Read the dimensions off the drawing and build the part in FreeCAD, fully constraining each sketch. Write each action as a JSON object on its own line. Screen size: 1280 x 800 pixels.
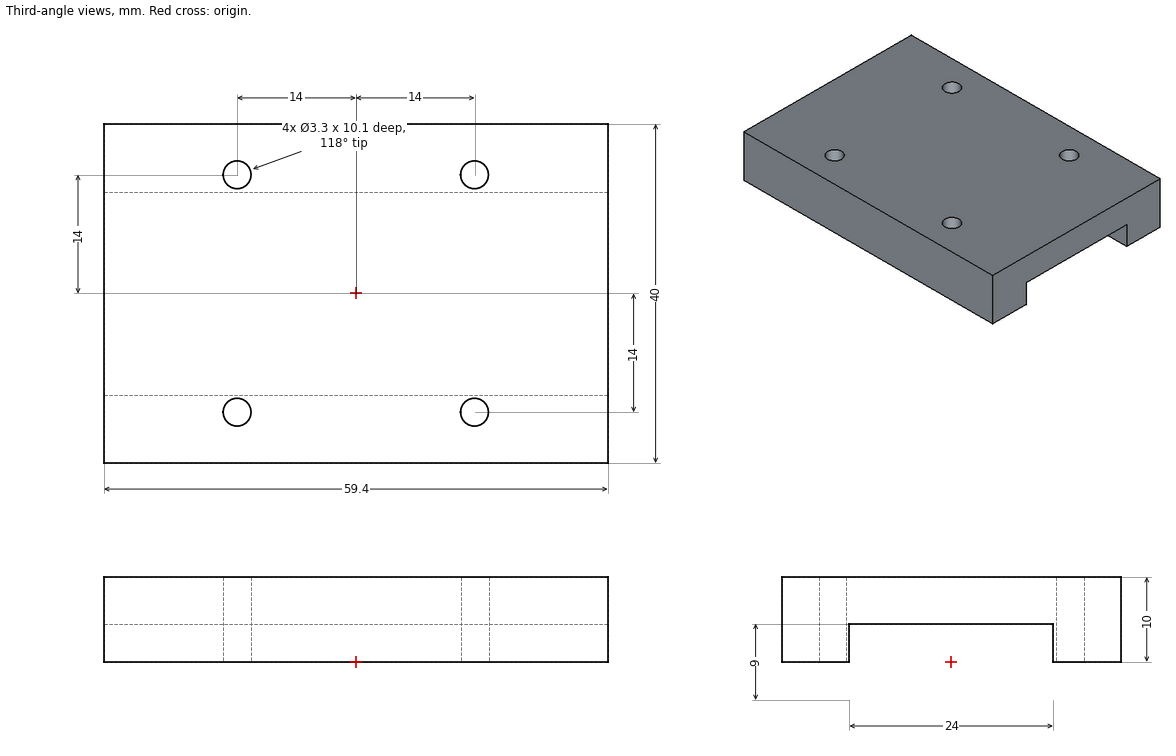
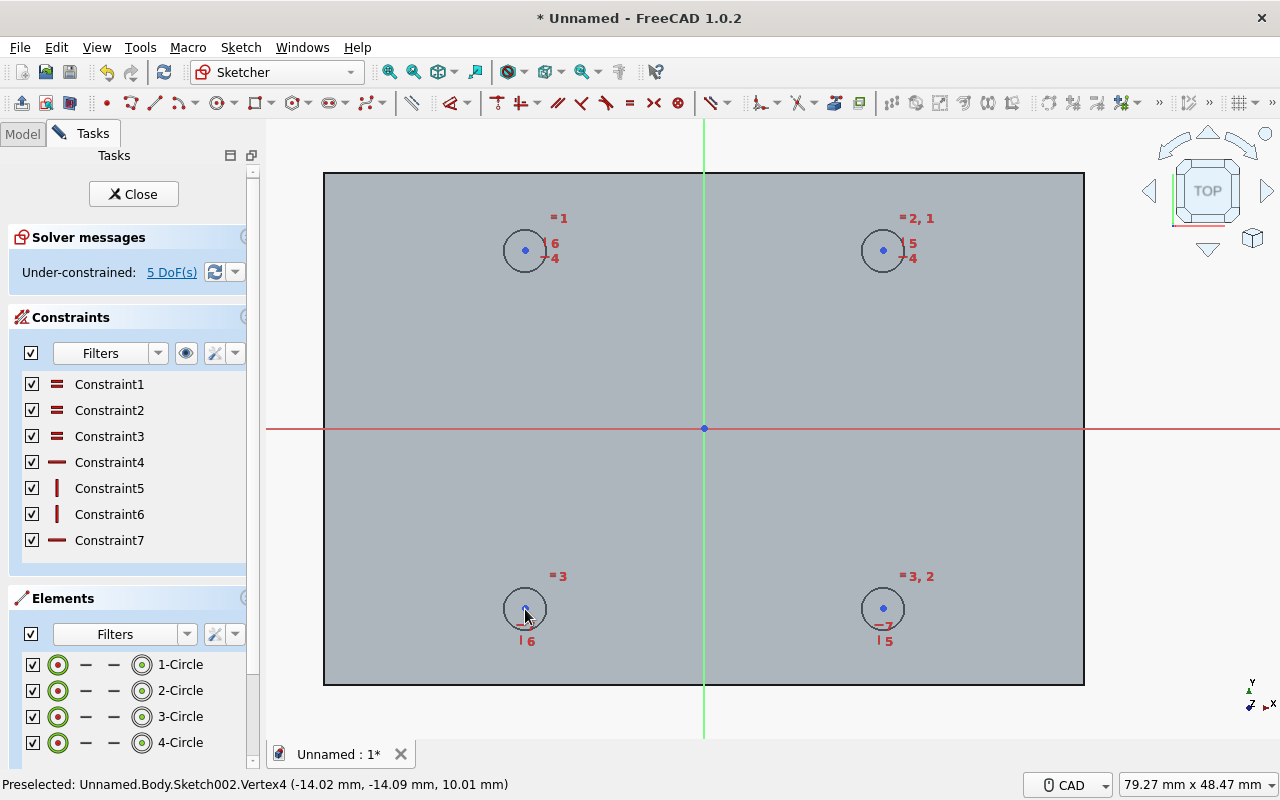
{"action": "key", "text": "d"}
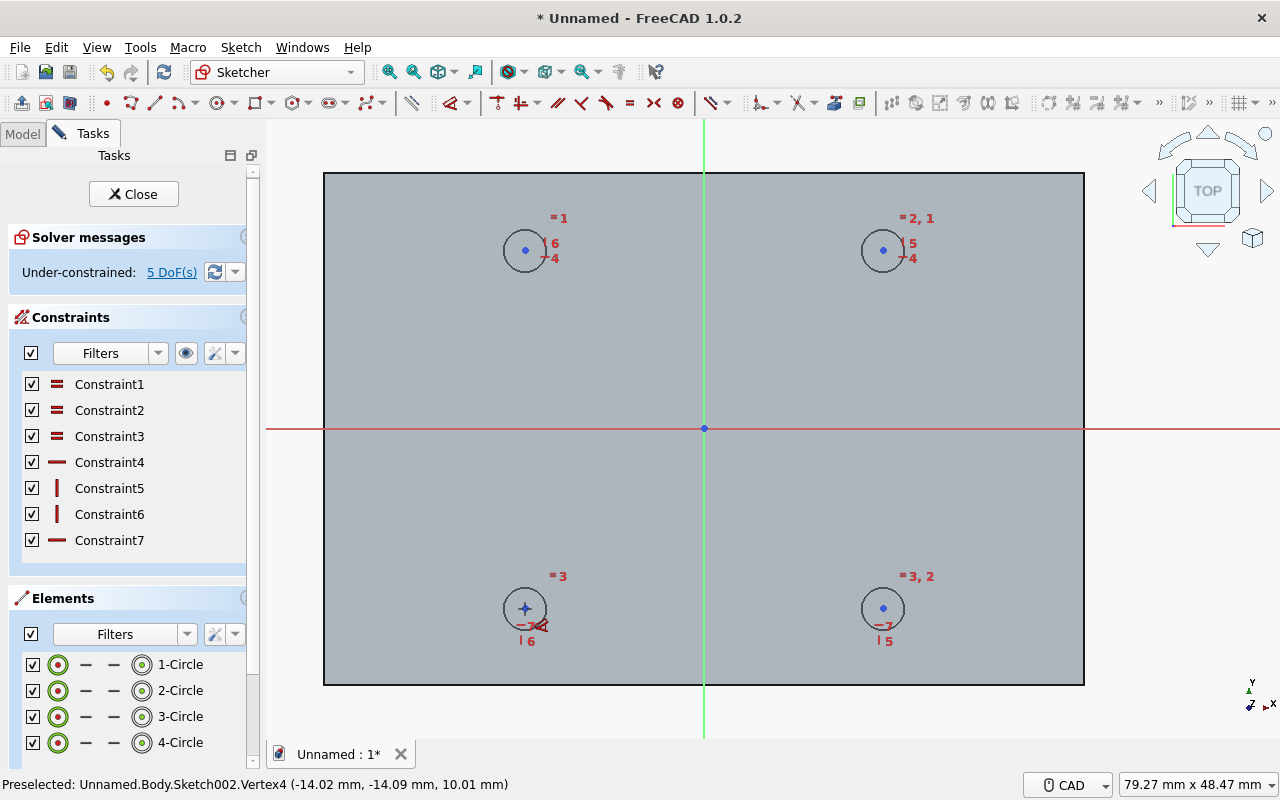
{"action": "left_click", "coordinate": [540, 236]}
{"action": "left_click", "coordinate": [563, 213]}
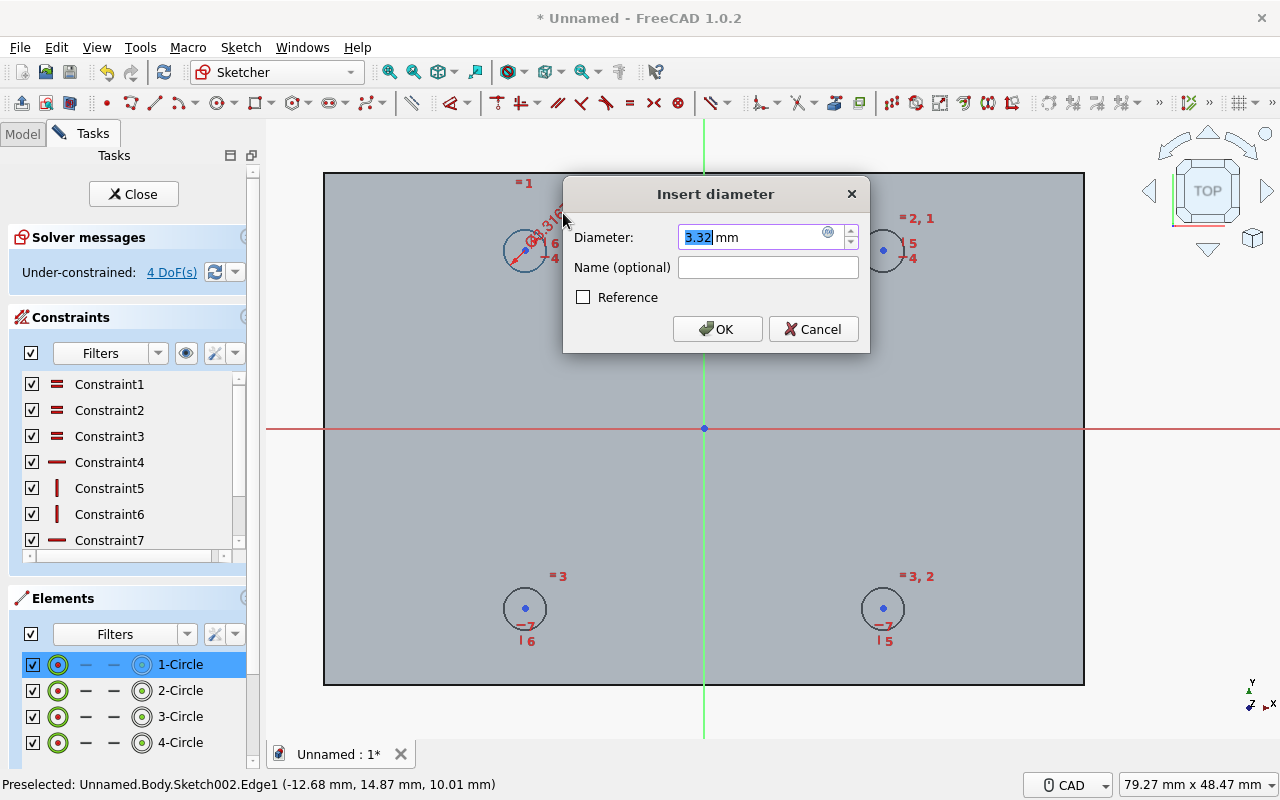
{"action": "type", "text": "3.3"}
{"action": "key", "text": "Return"}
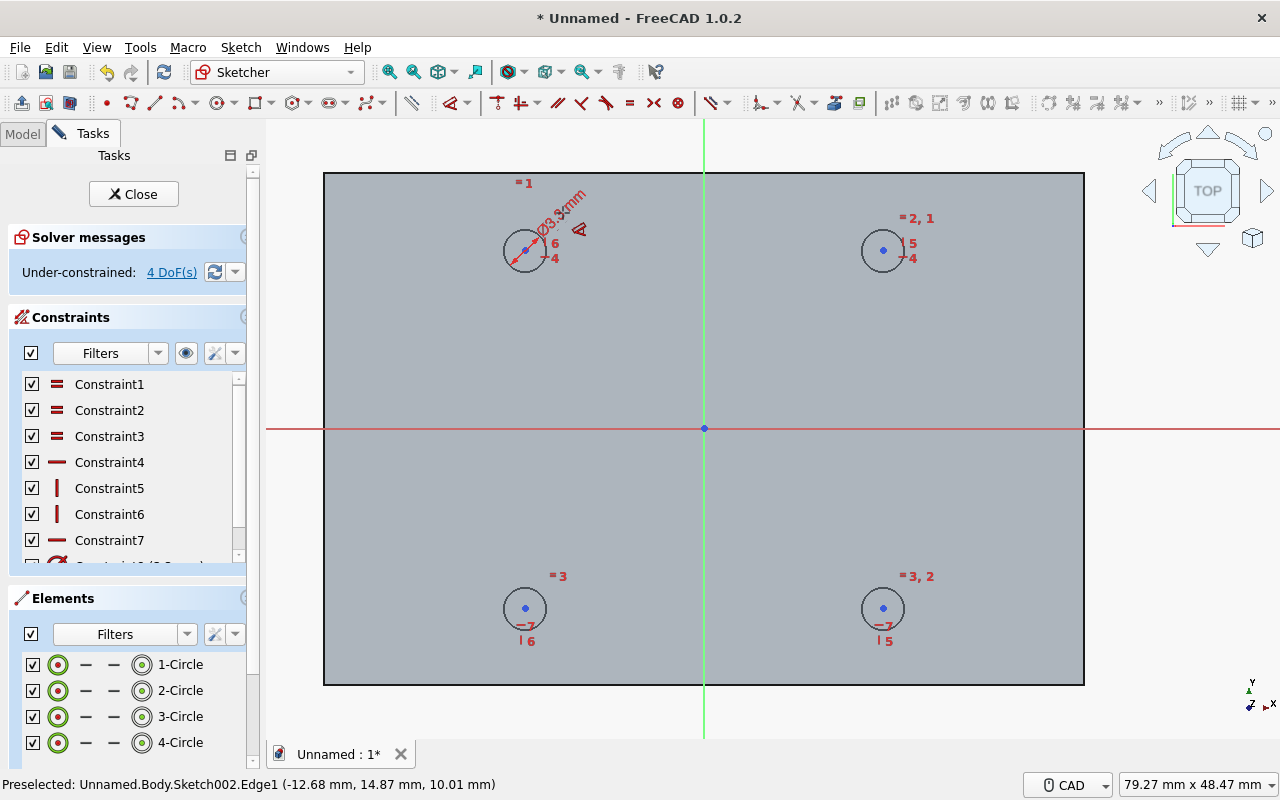
{"action": "left_click", "coordinate": [525, 251]}
{"action": "left_click", "coordinate": [656, 217]}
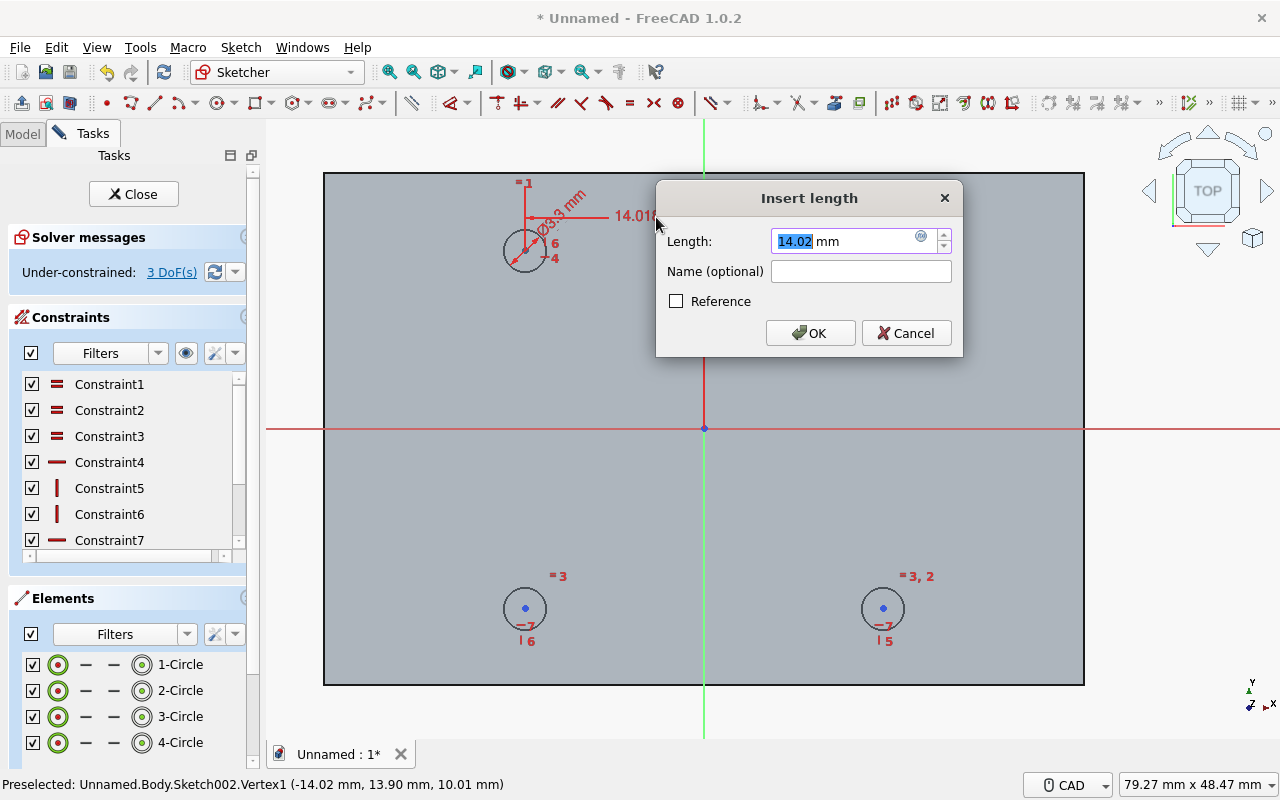
{"action": "type", "text": "14"}
{"action": "key", "text": "Return"}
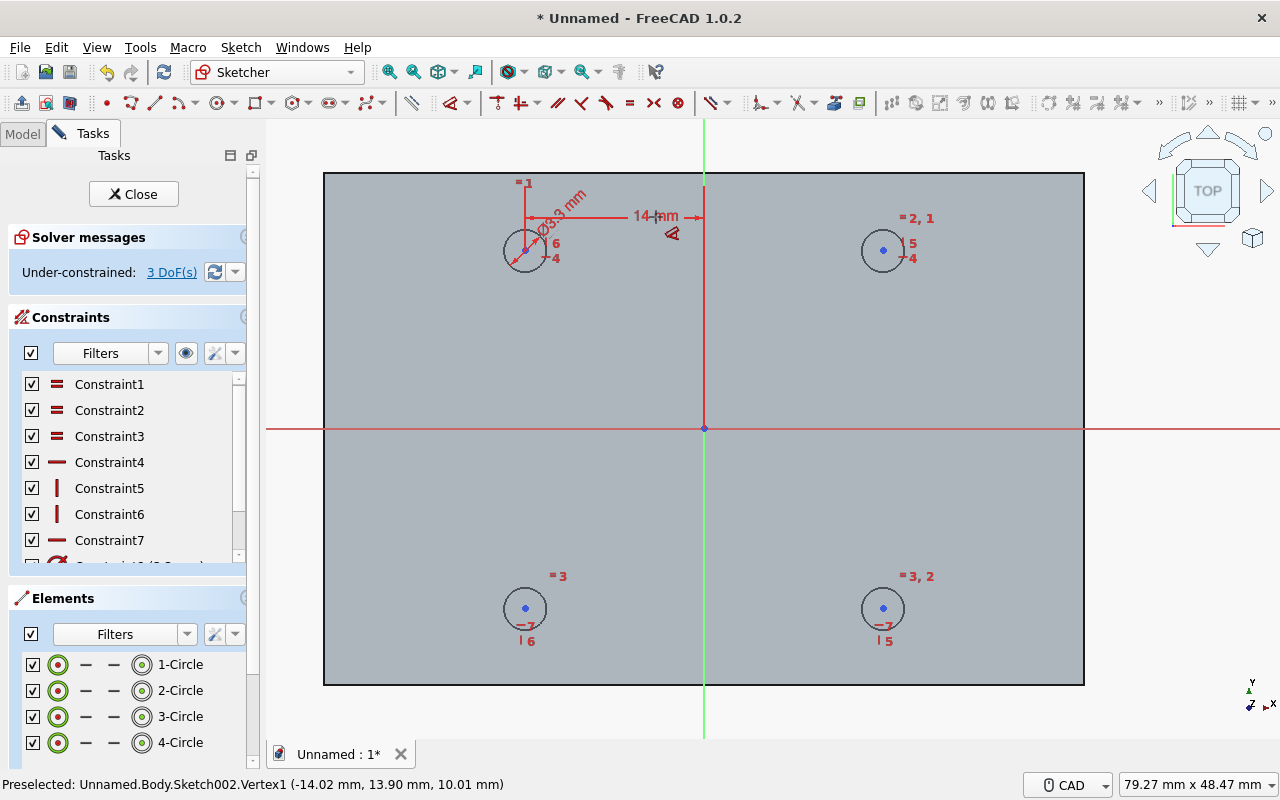
{"action": "left_click", "coordinate": [525, 251]}
{"action": "left_click", "coordinate": [491, 340]}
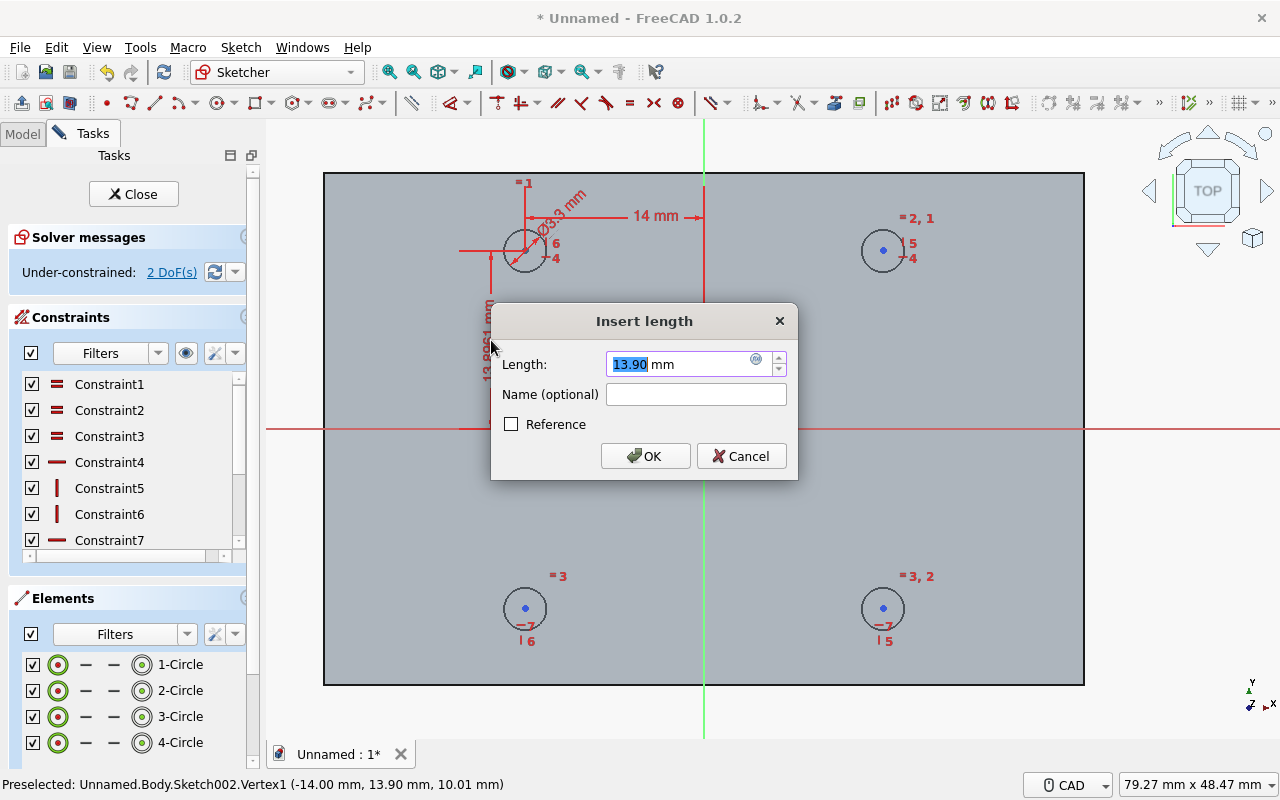
{"action": "type", "text": "14"}
{"action": "key", "text": "Return"}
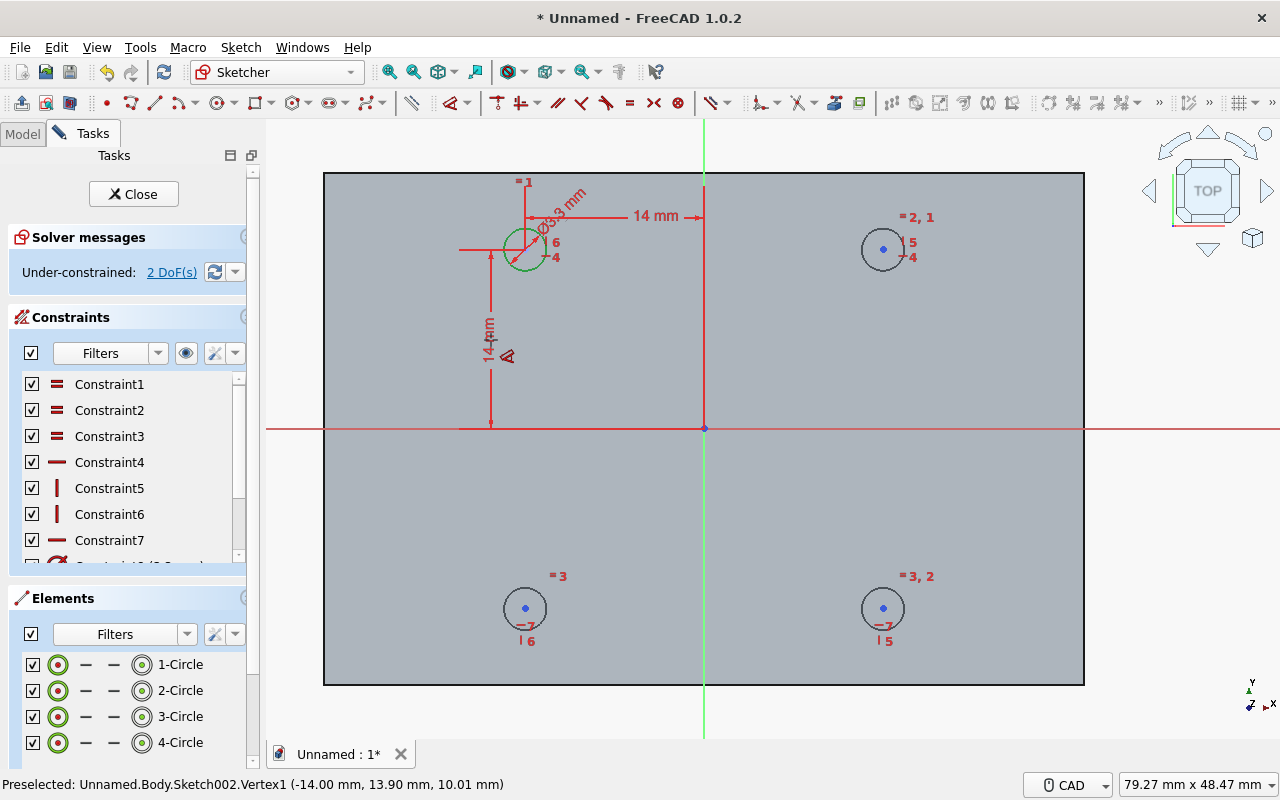
{"action": "left_click", "coordinate": [883, 250]}
{"action": "left_click", "coordinate": [794, 216]}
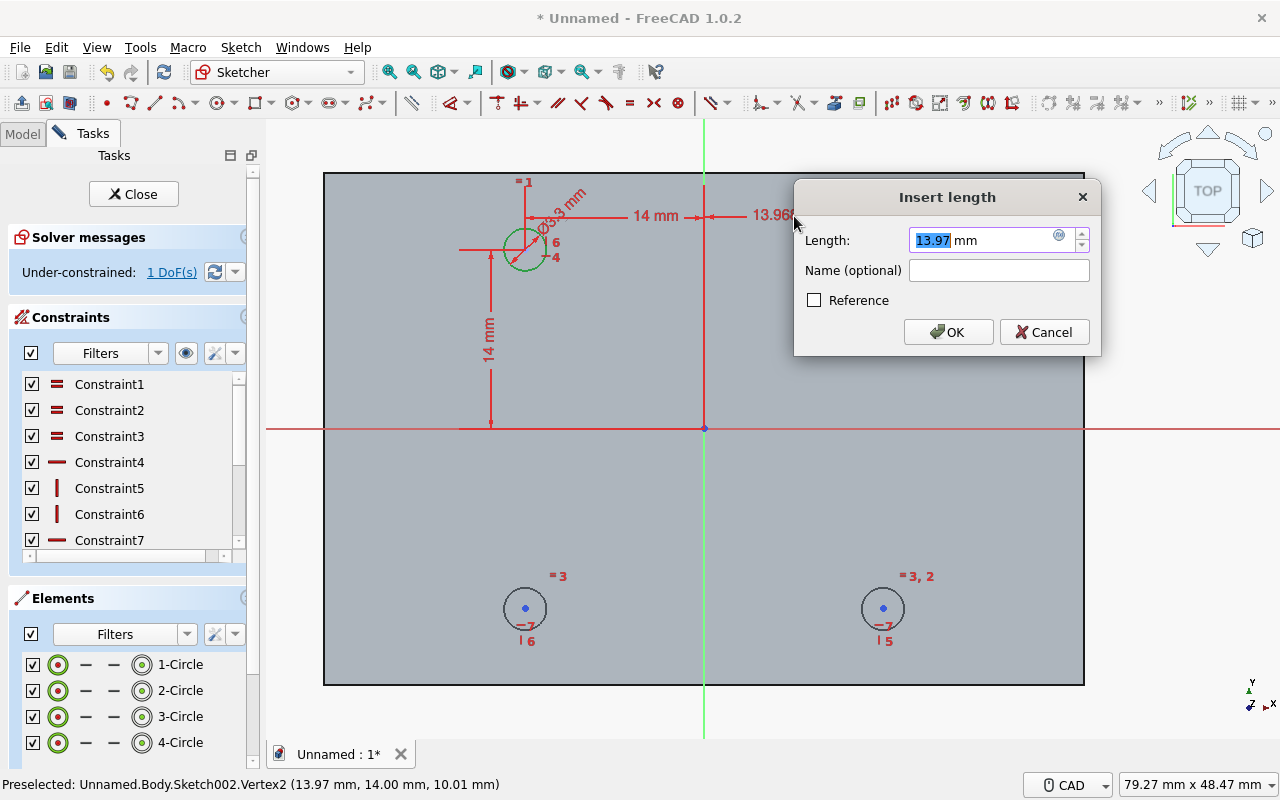
{"action": "type", "text": "14"}
{"action": "key", "text": "Return"}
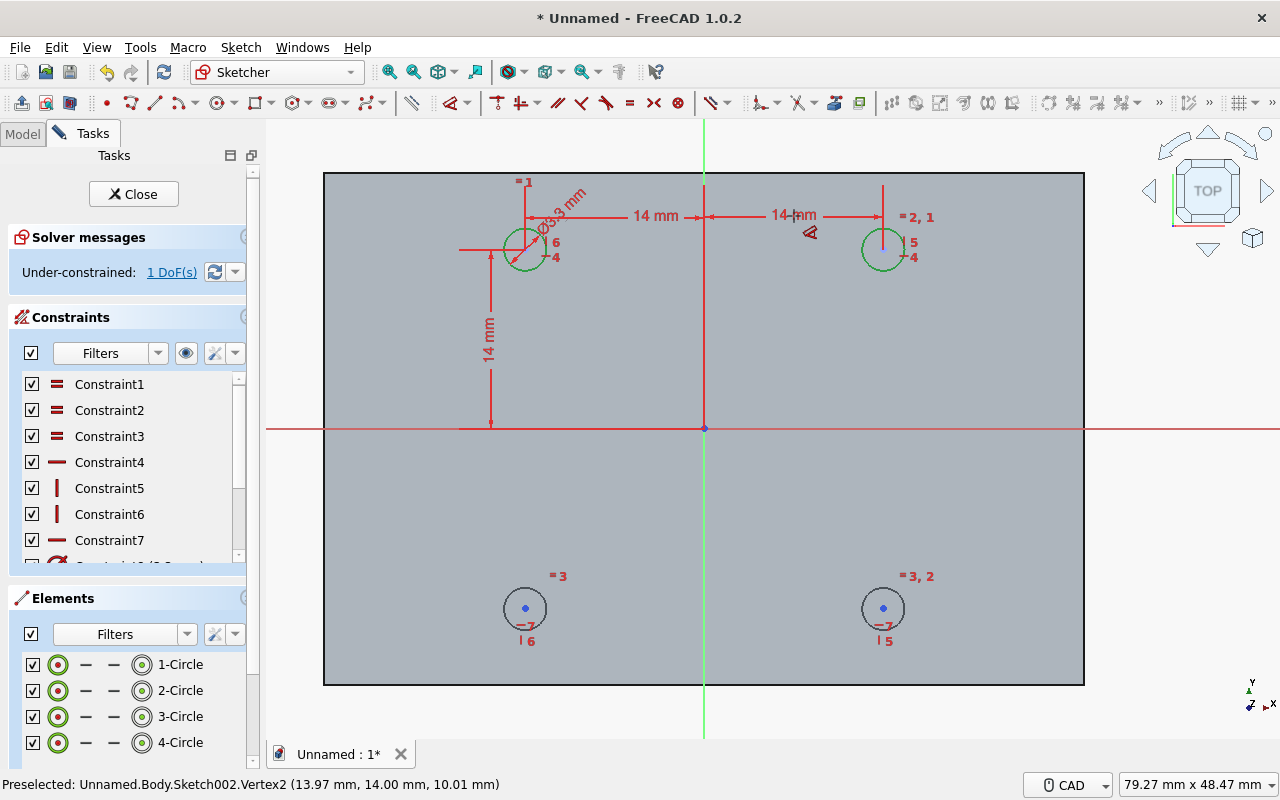
{"action": "left_click", "coordinate": [883, 609]}
{"action": "left_click", "coordinate": [917, 519]}